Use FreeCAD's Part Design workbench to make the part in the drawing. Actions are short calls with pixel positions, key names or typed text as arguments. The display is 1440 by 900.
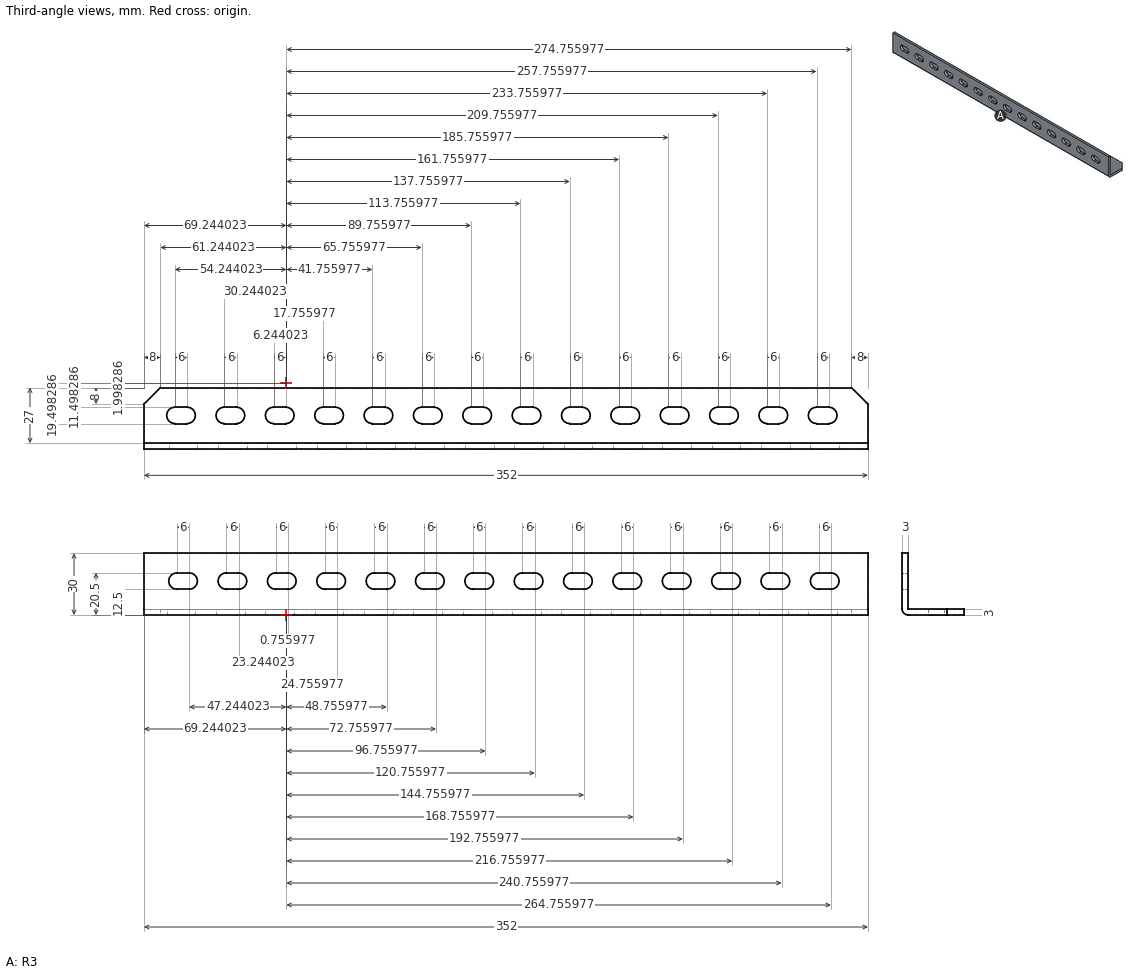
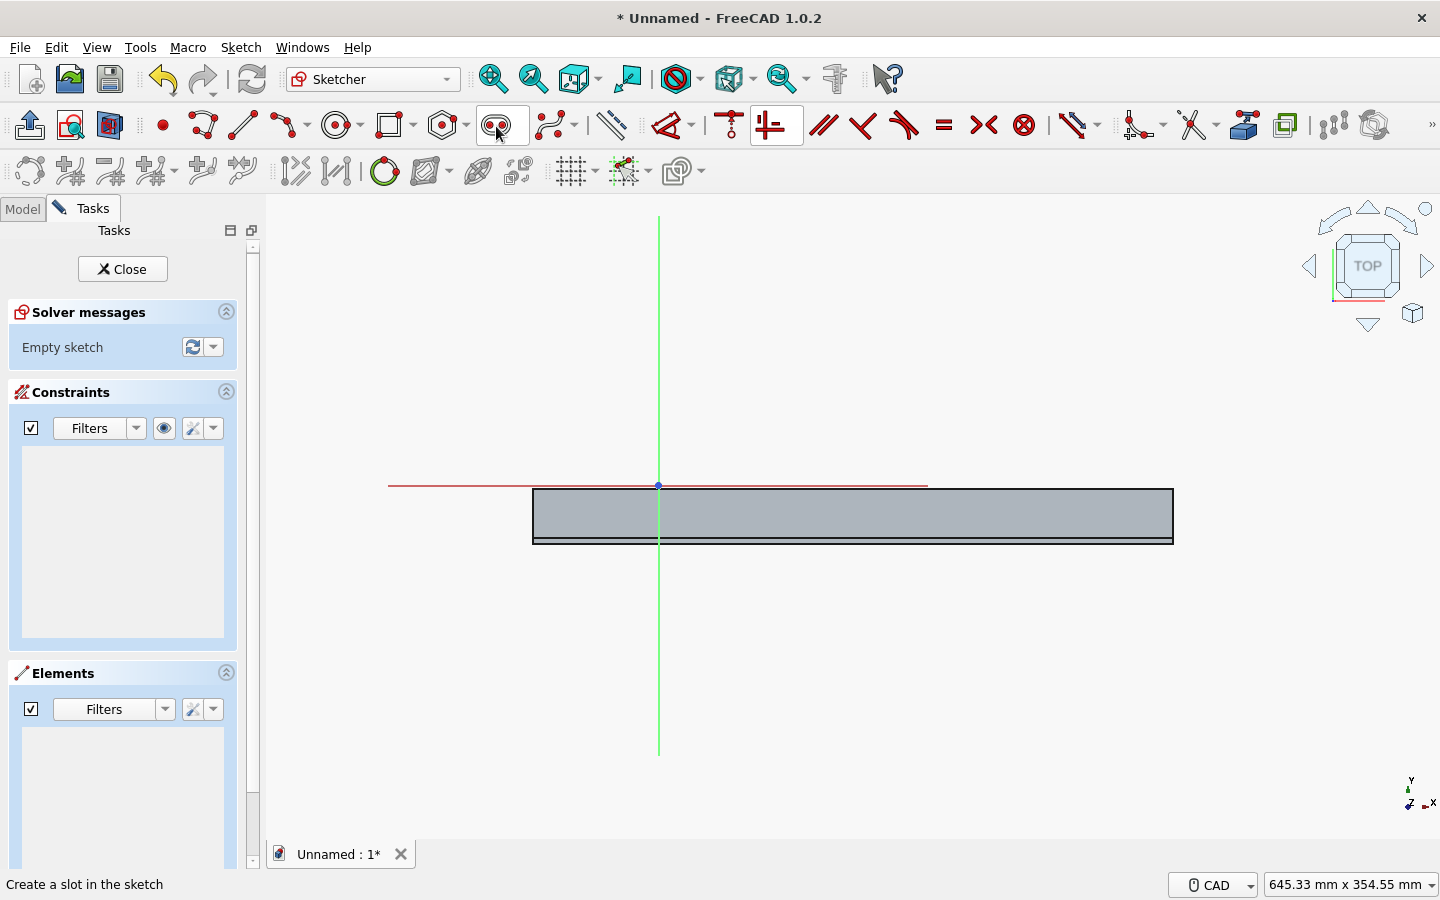
scroll(560, 514, up, 6)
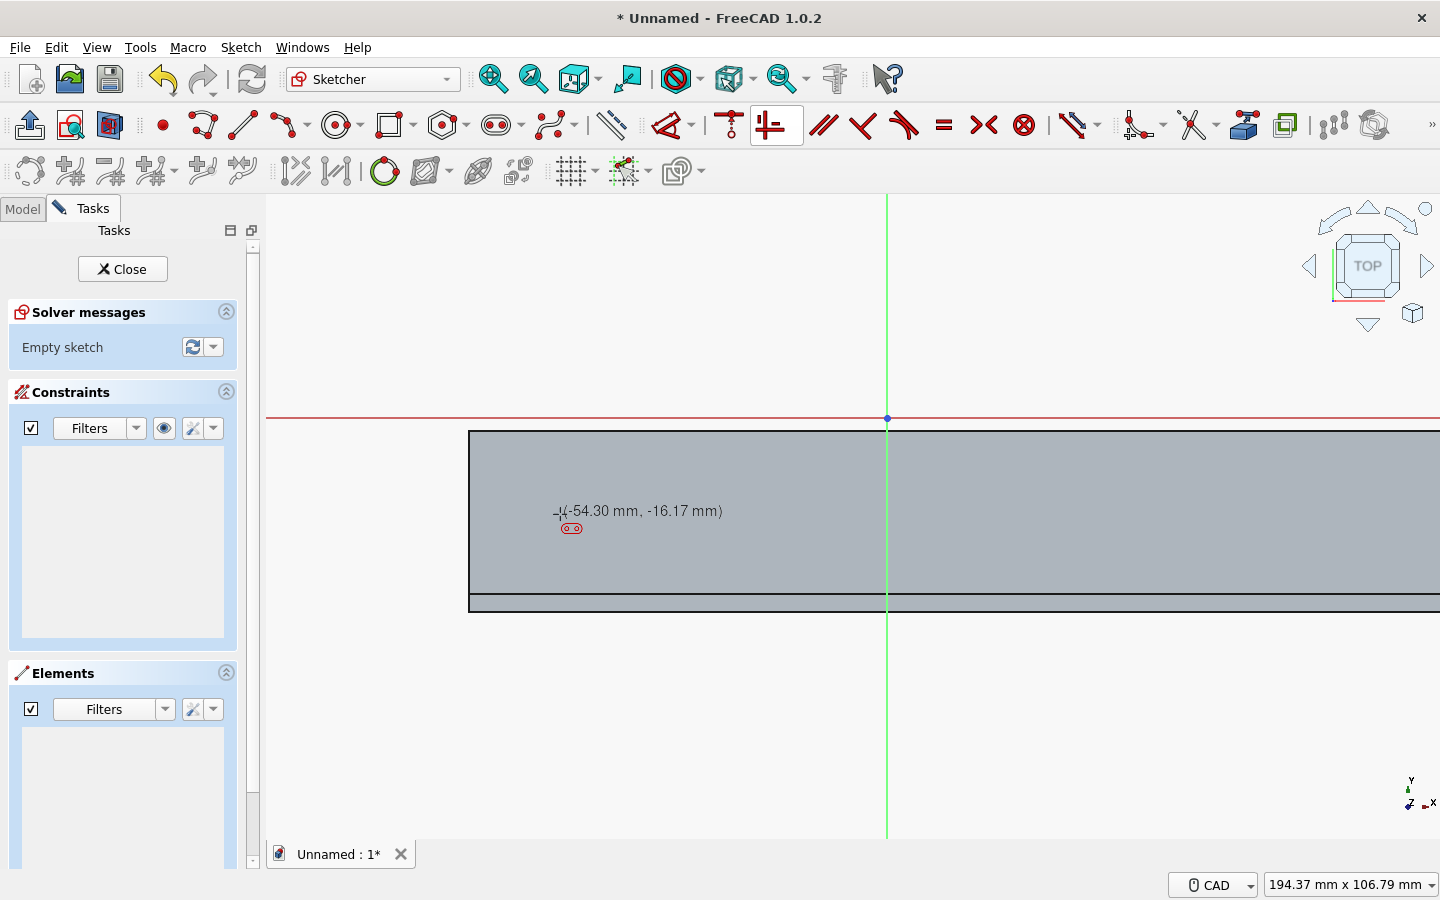
click(560, 512)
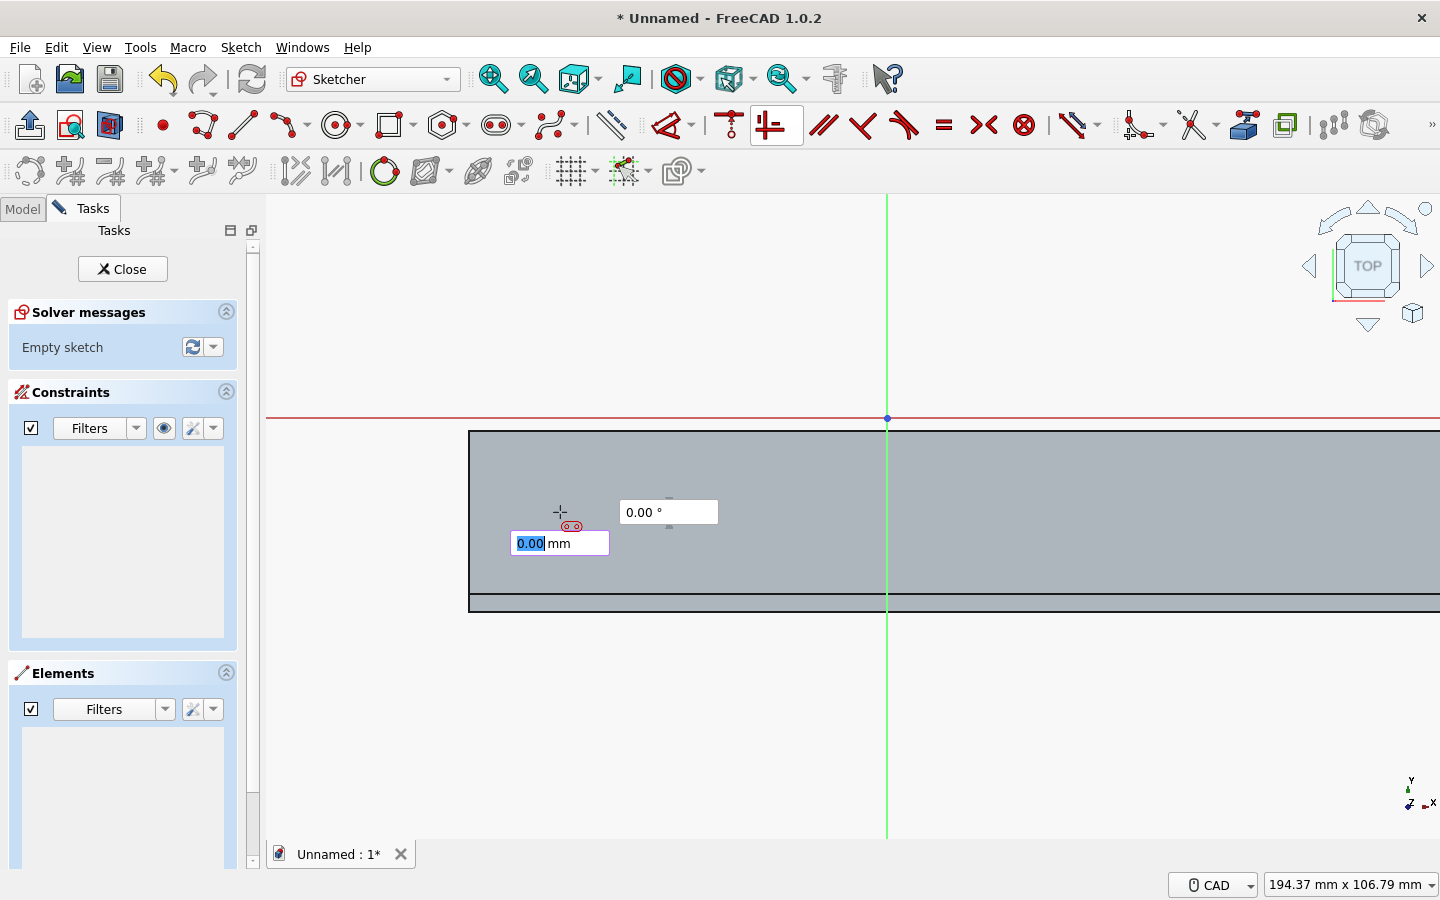
click(596, 512)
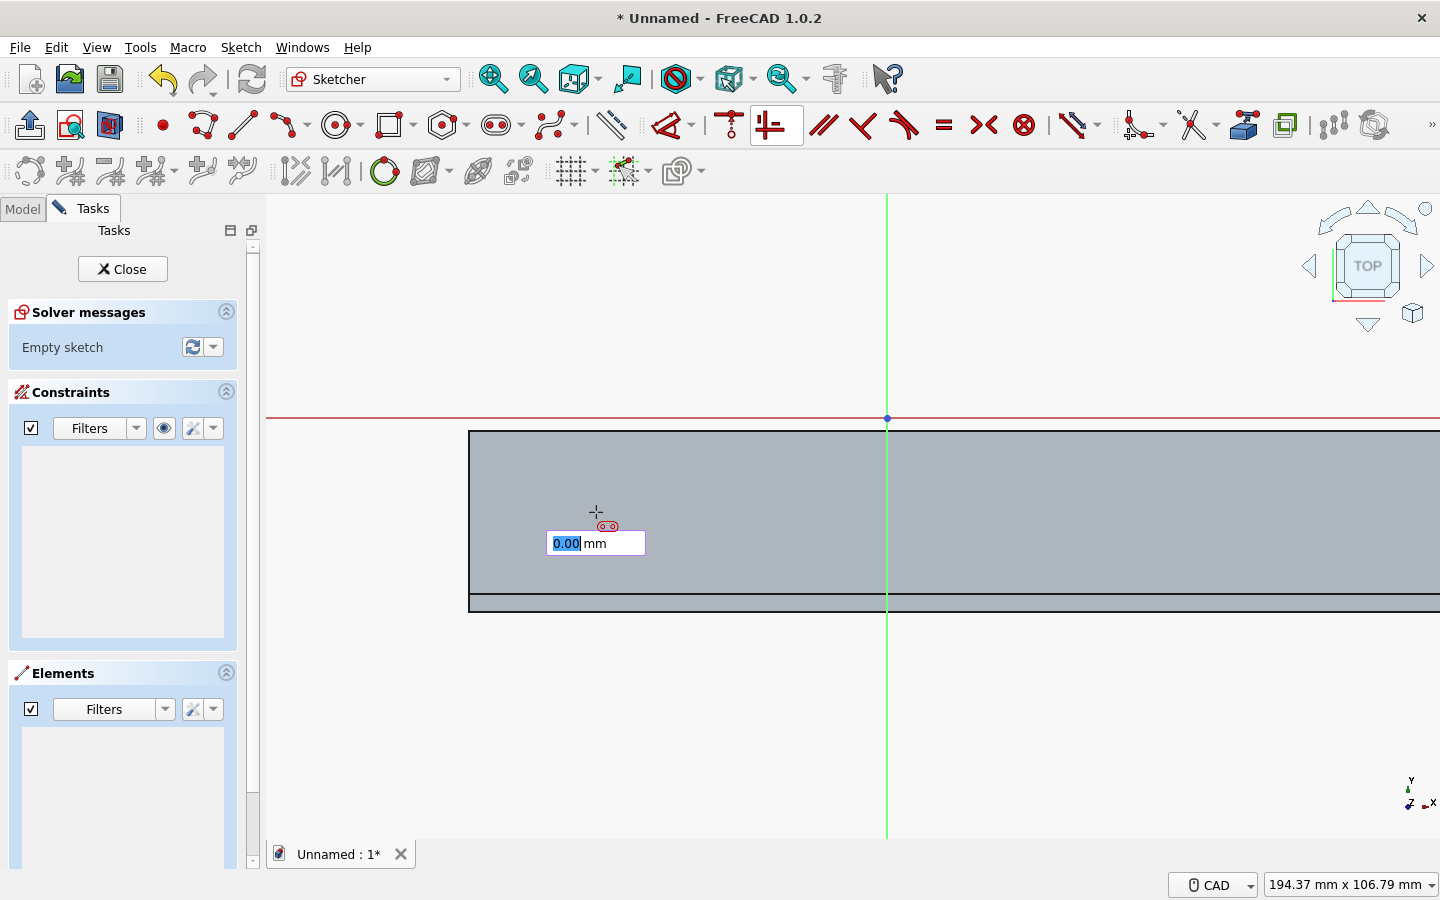
click(578, 488)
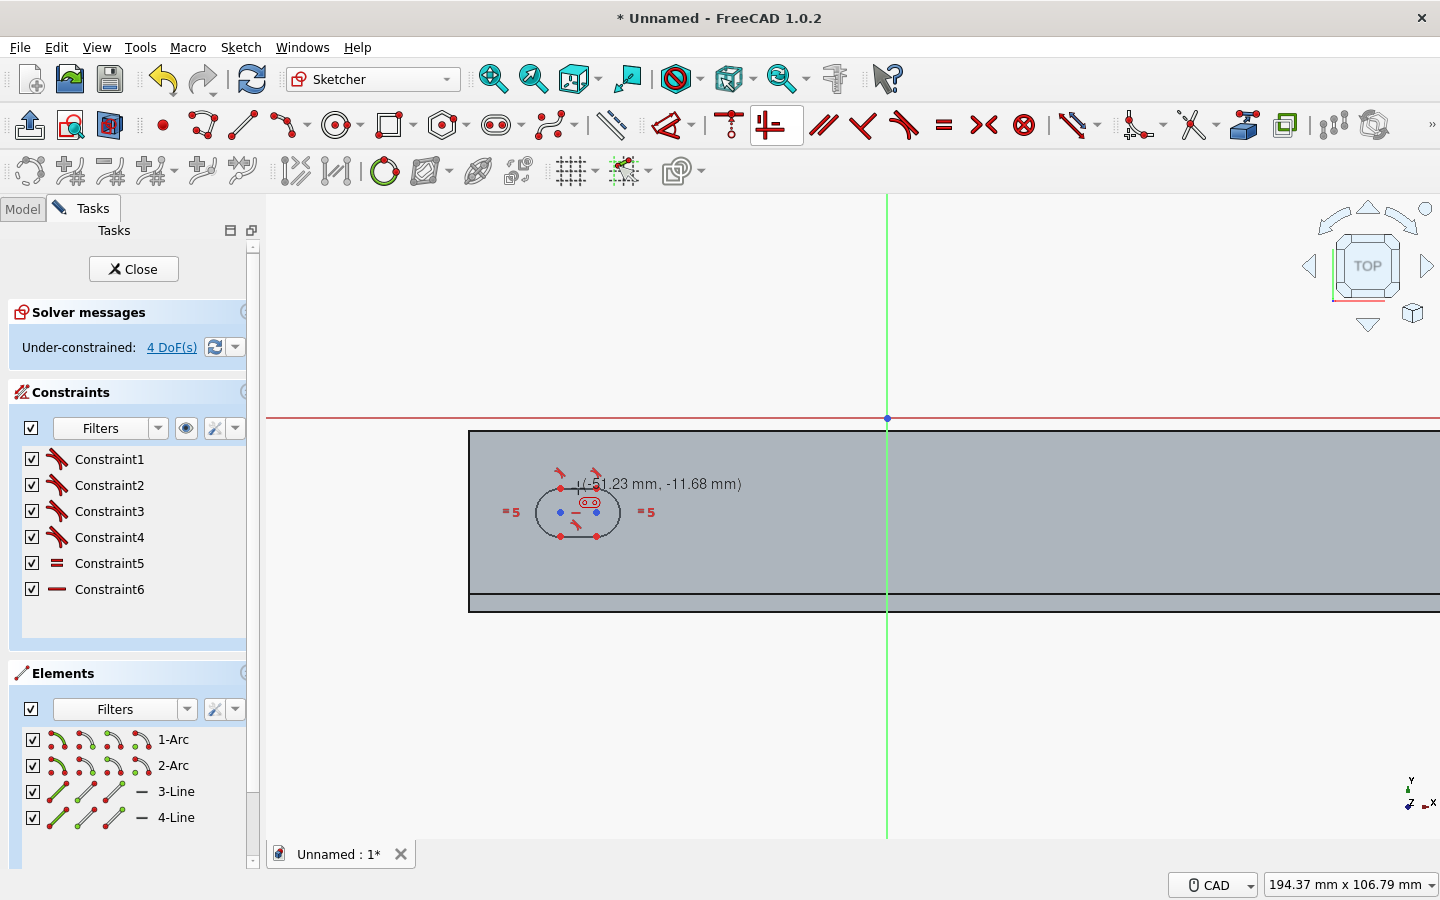
click(705, 512)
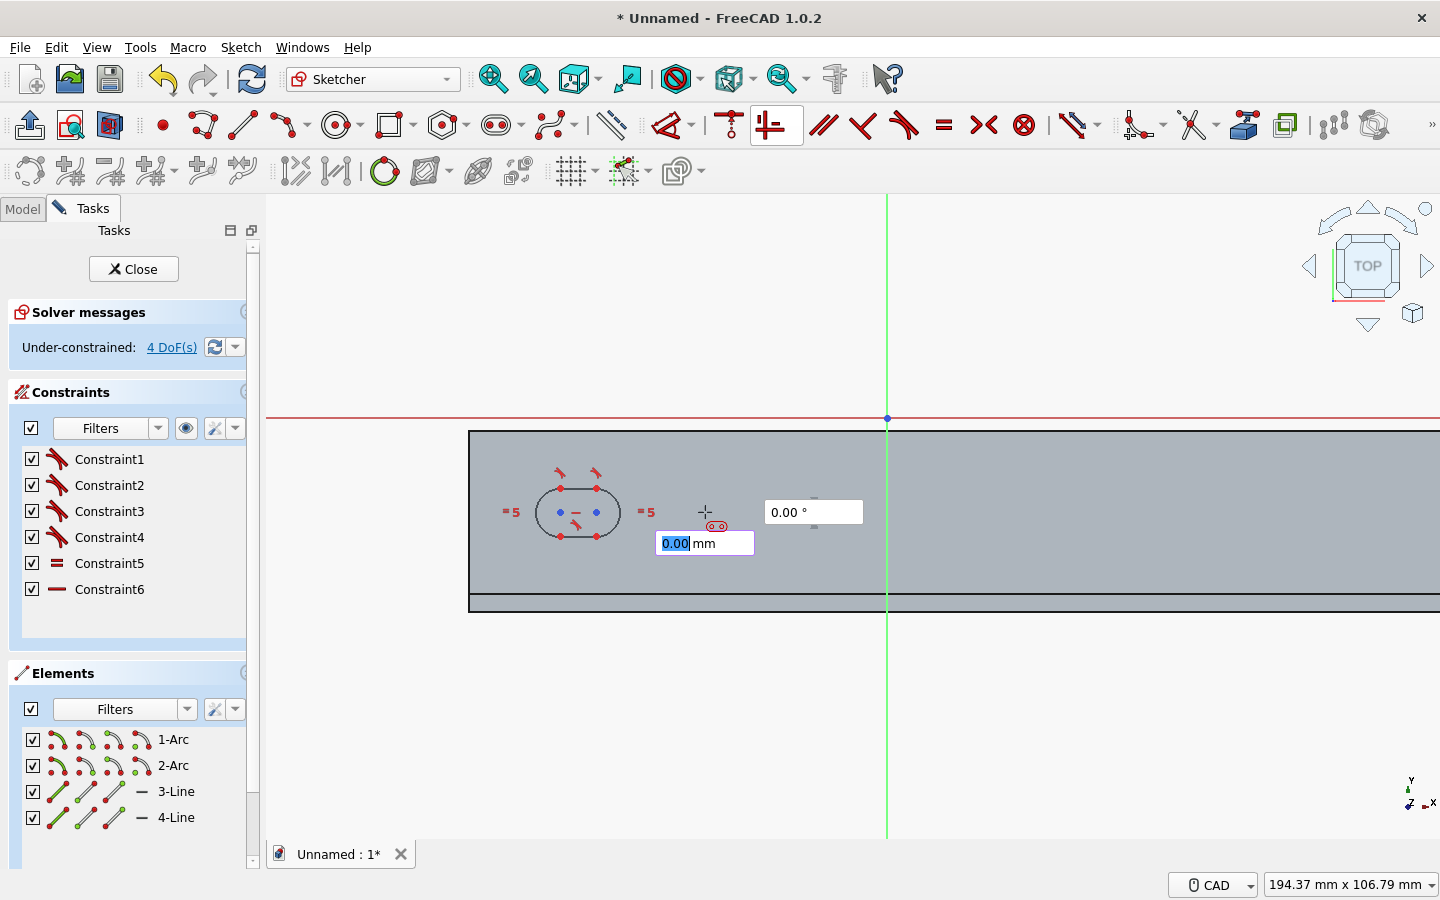
click(741, 512)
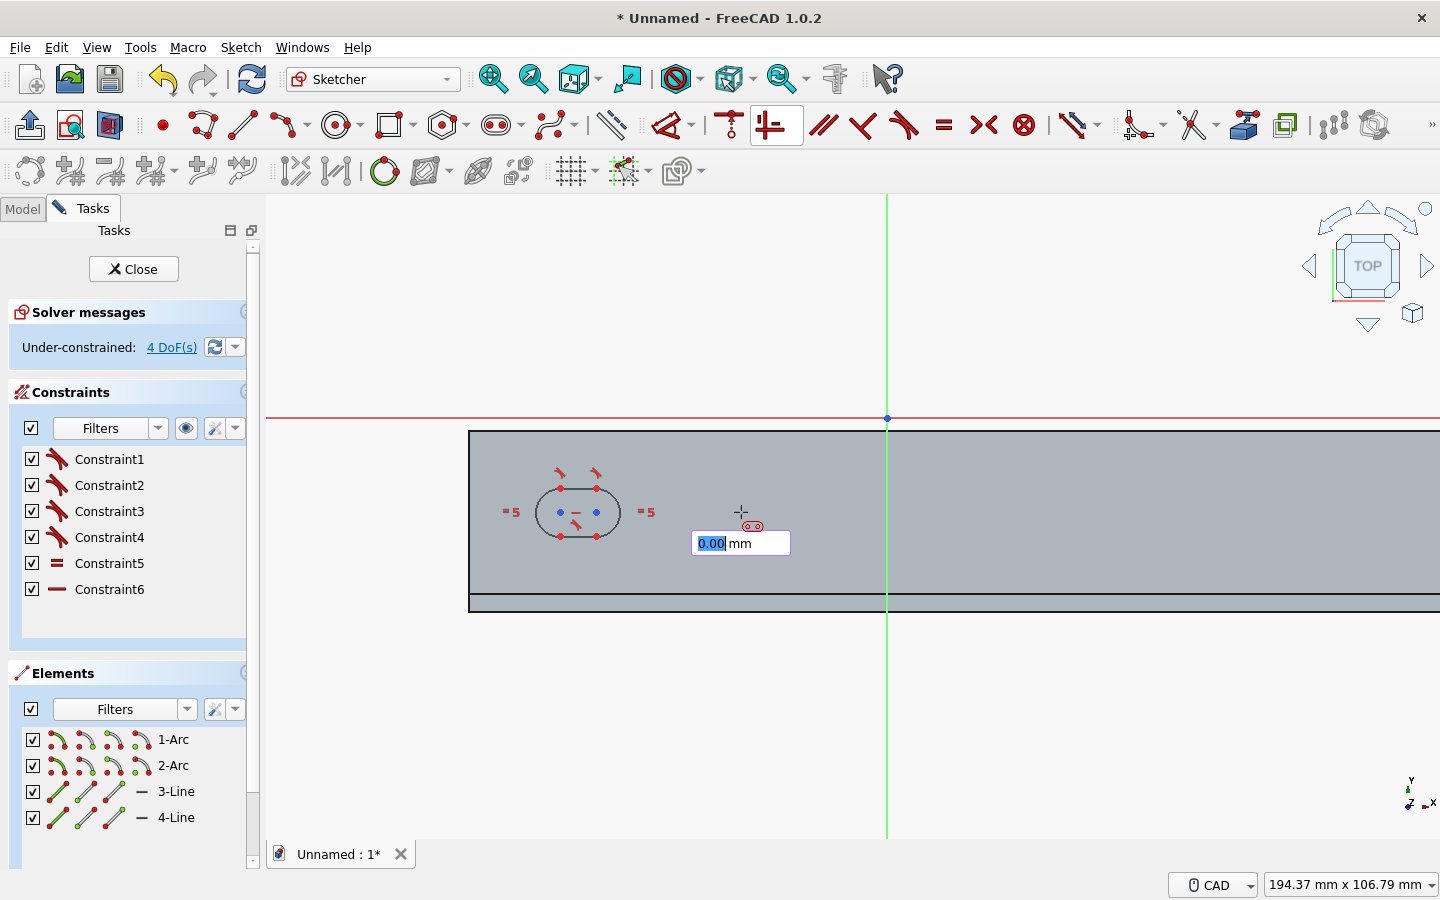
click(723, 488)